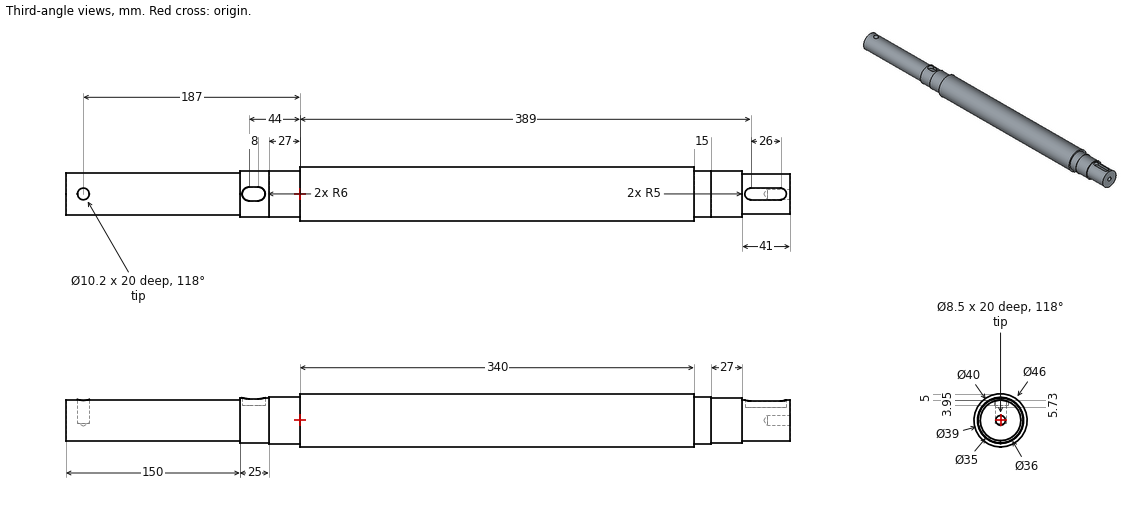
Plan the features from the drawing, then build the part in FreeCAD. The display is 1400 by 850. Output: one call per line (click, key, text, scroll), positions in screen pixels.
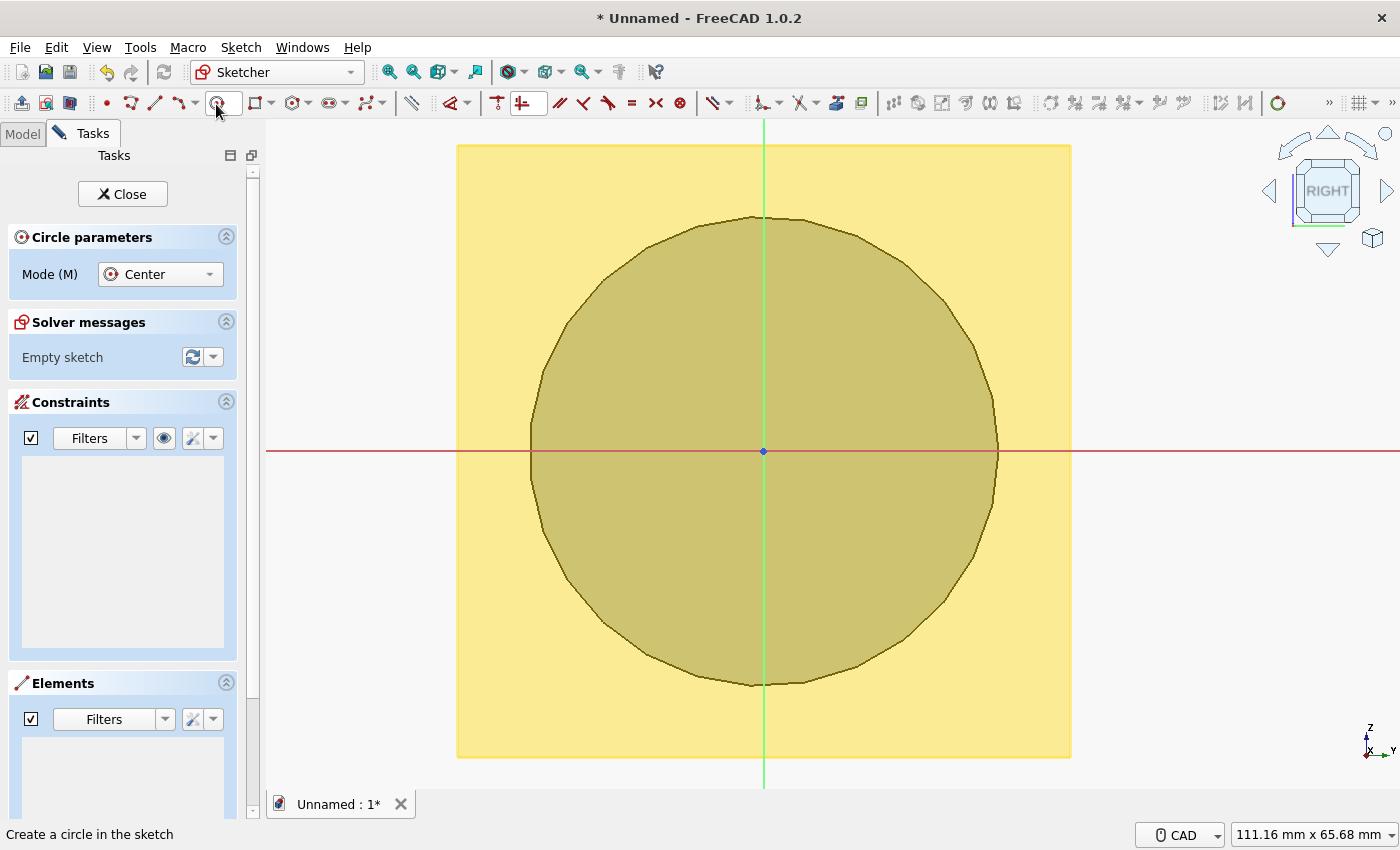
click(764, 451)
click(908, 307)
key(Escape)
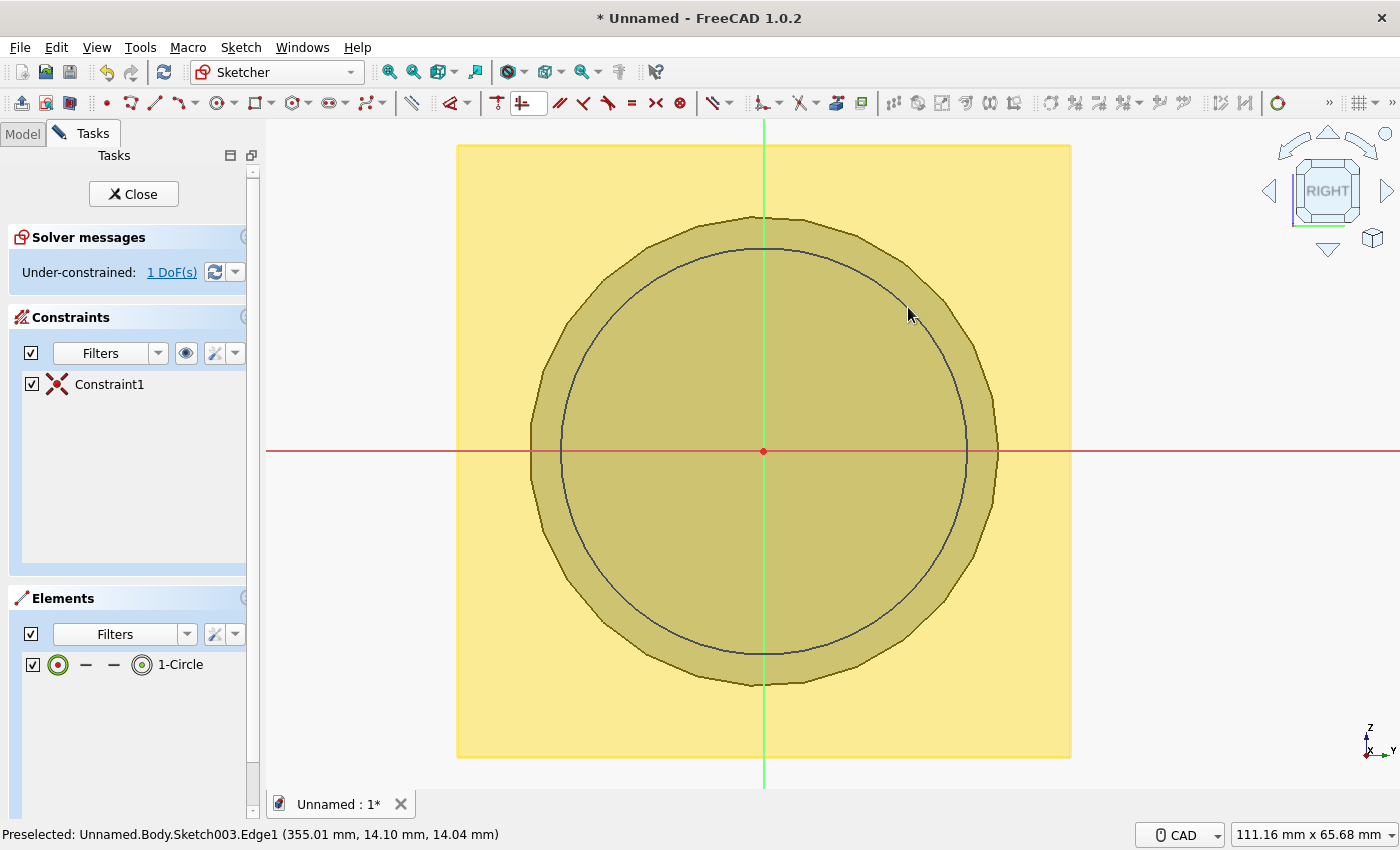
click(450, 104)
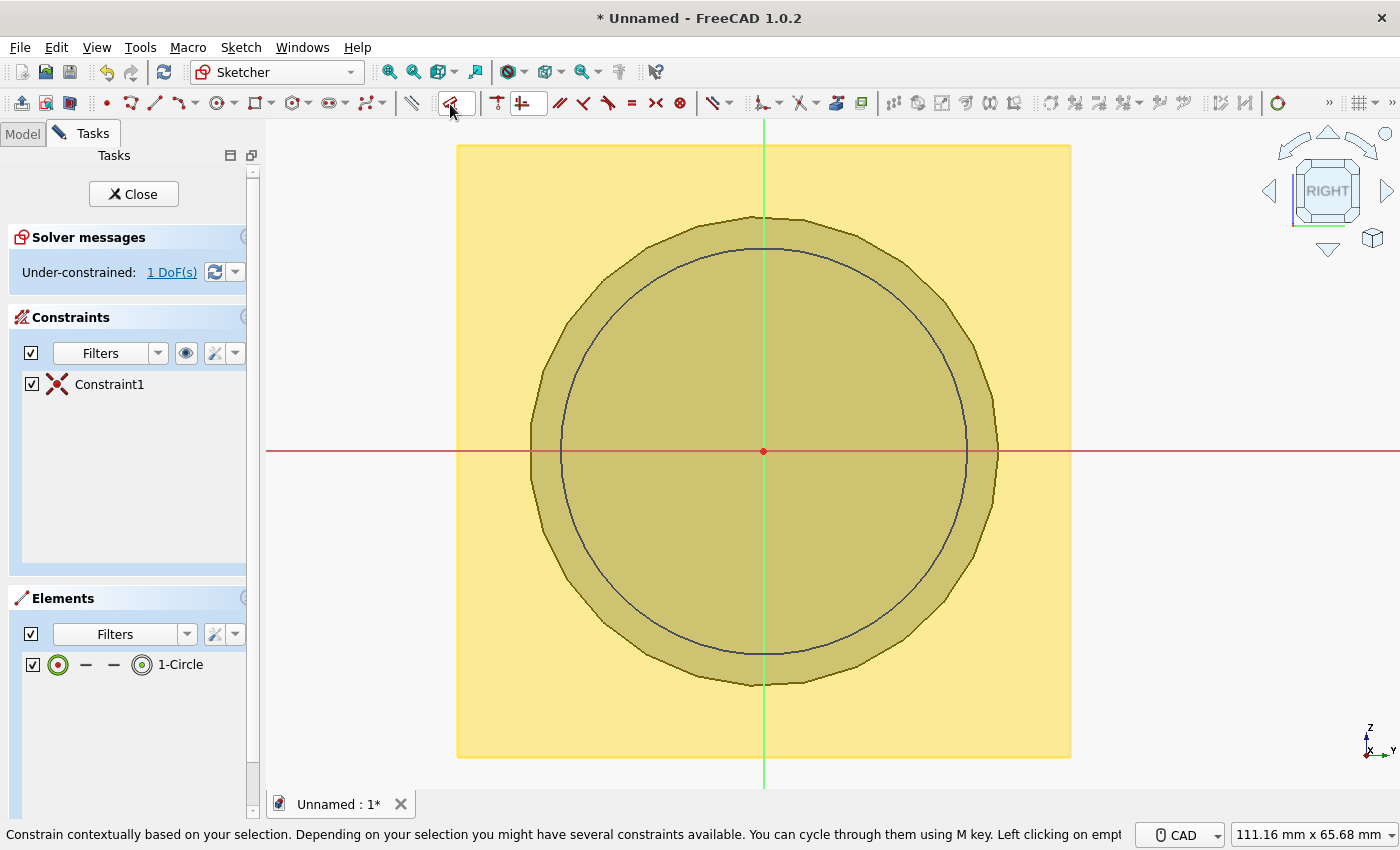
click(907, 307)
click(930, 284)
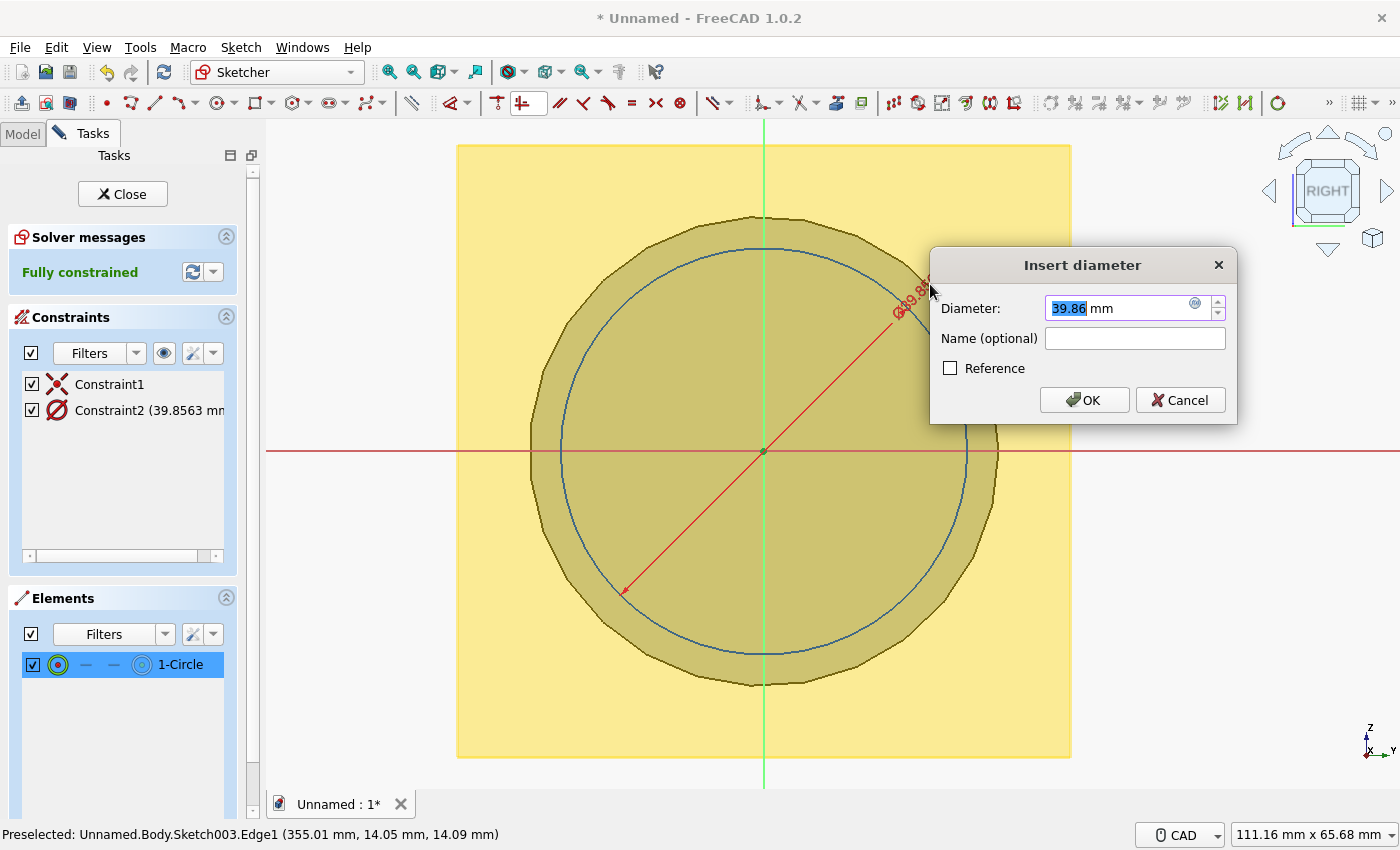
text(40)
key(Return)
key(Escape)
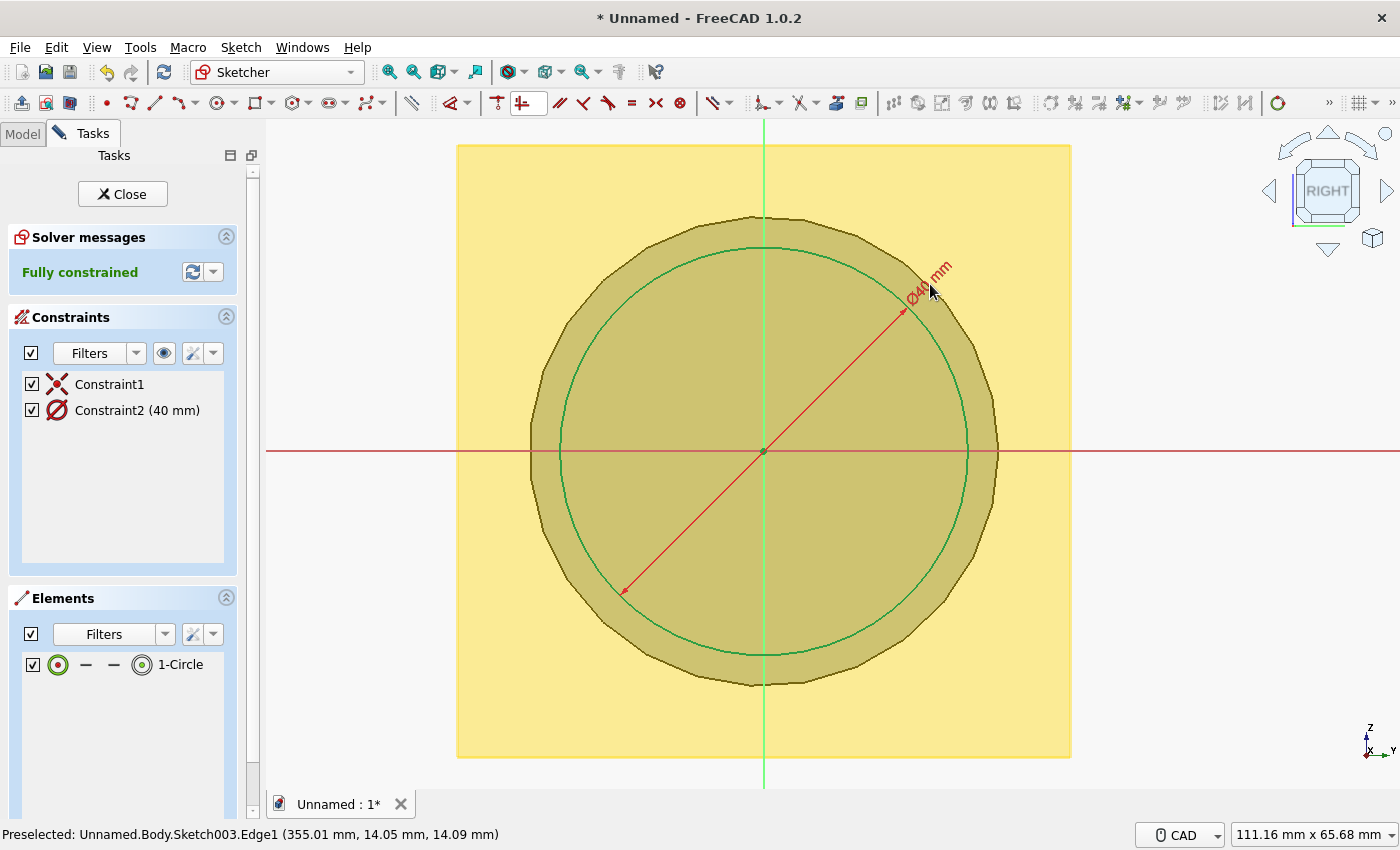
click(123, 194)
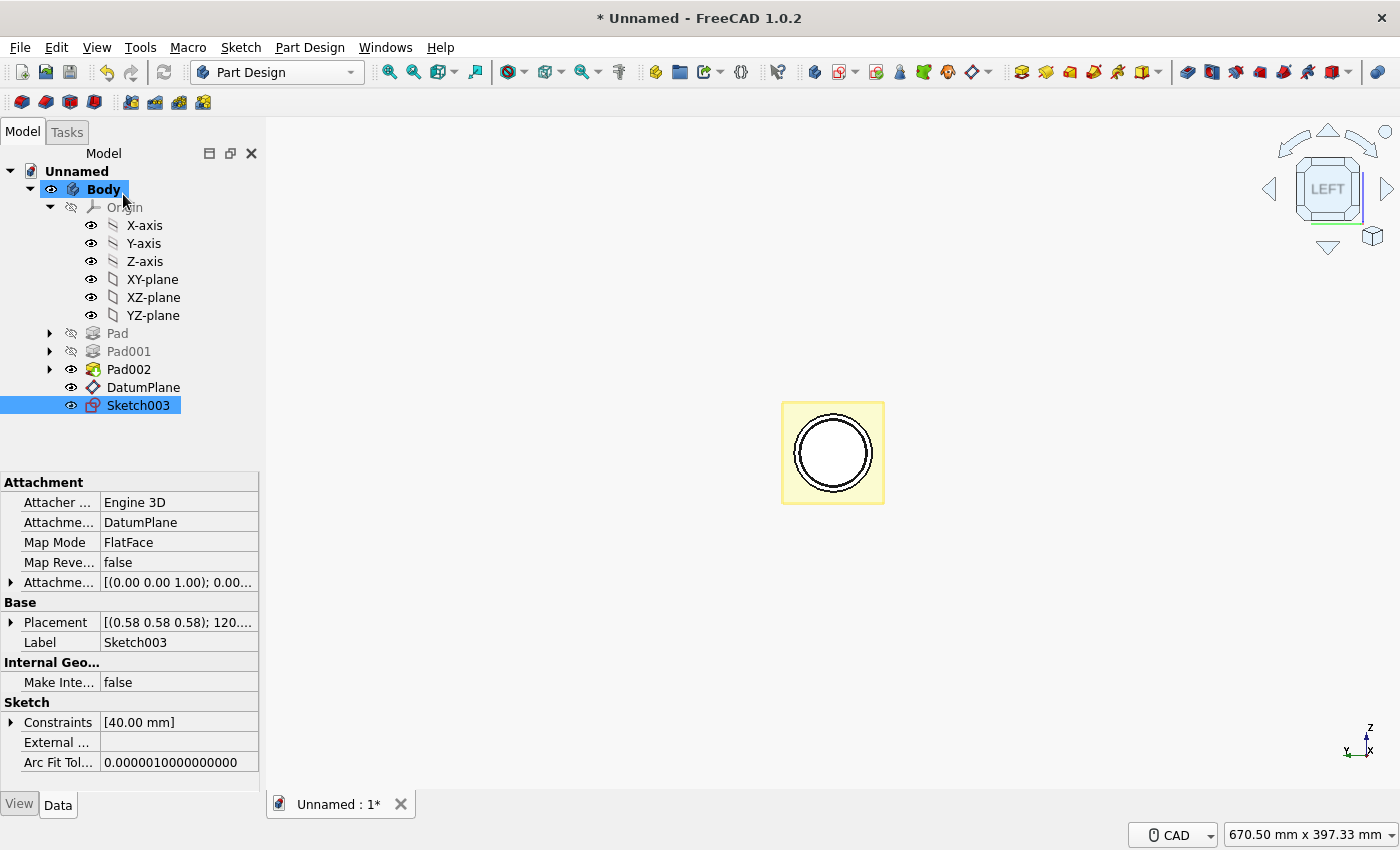
click(1022, 72)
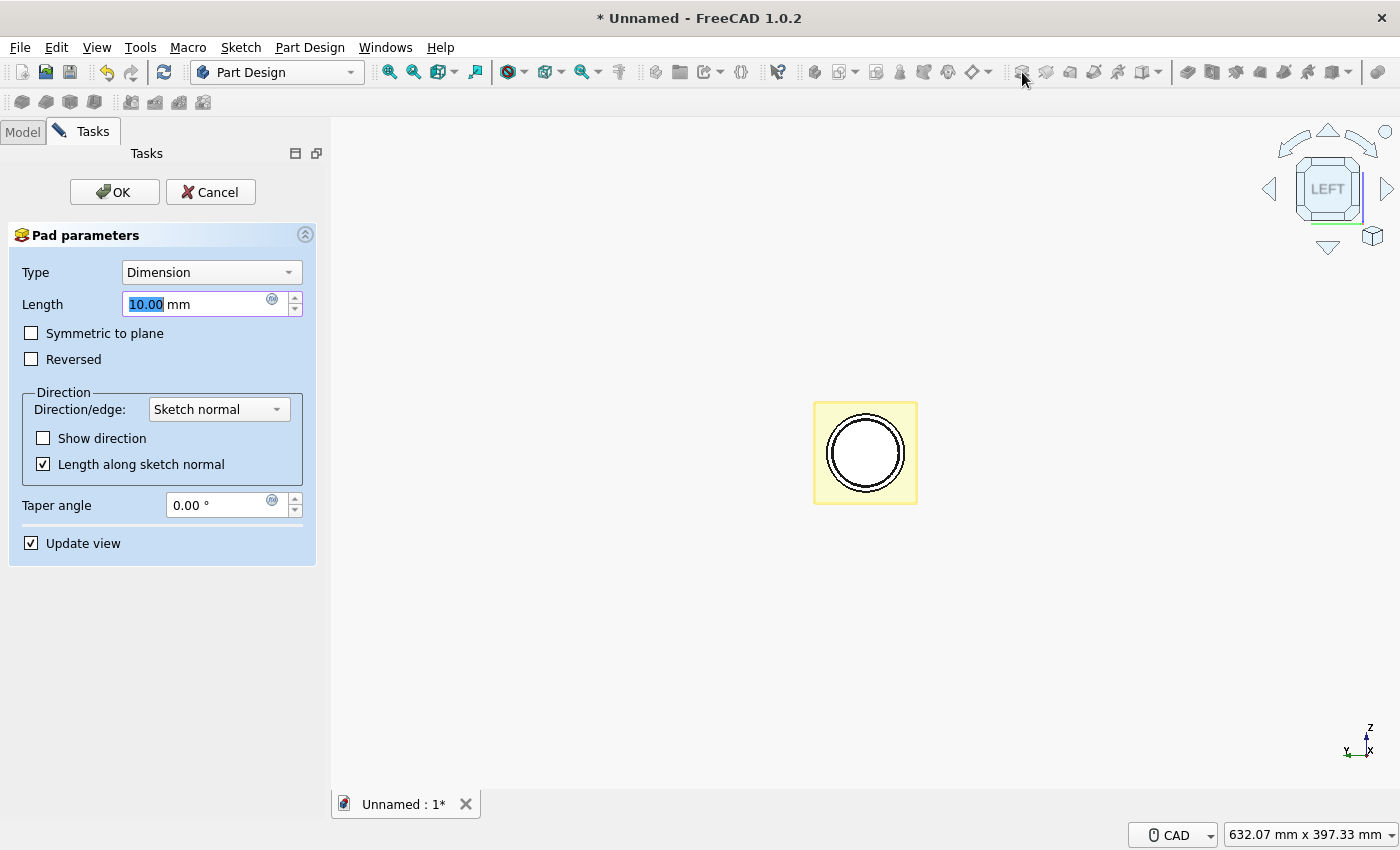
text(15)
key(Tab)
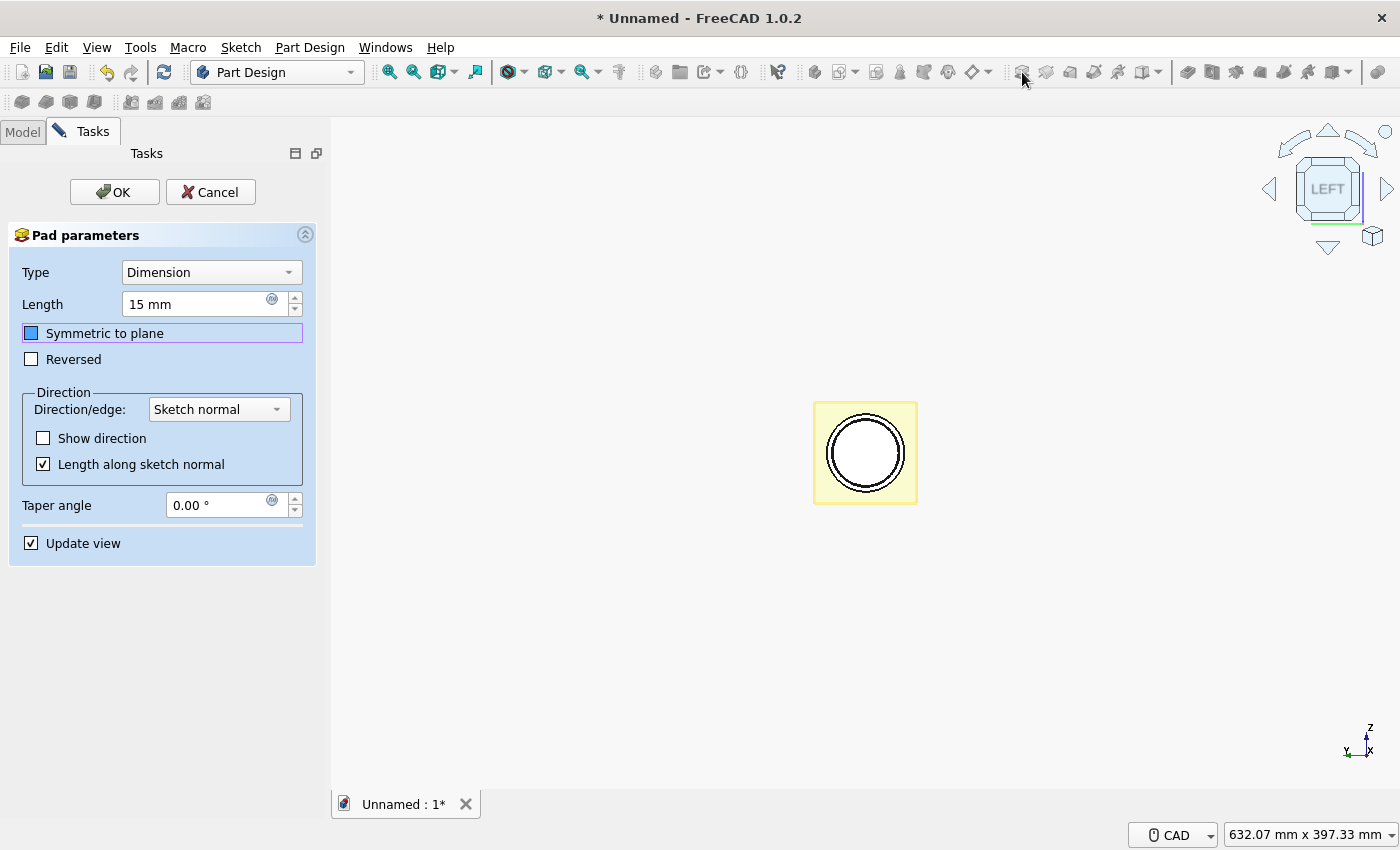
click(30, 359)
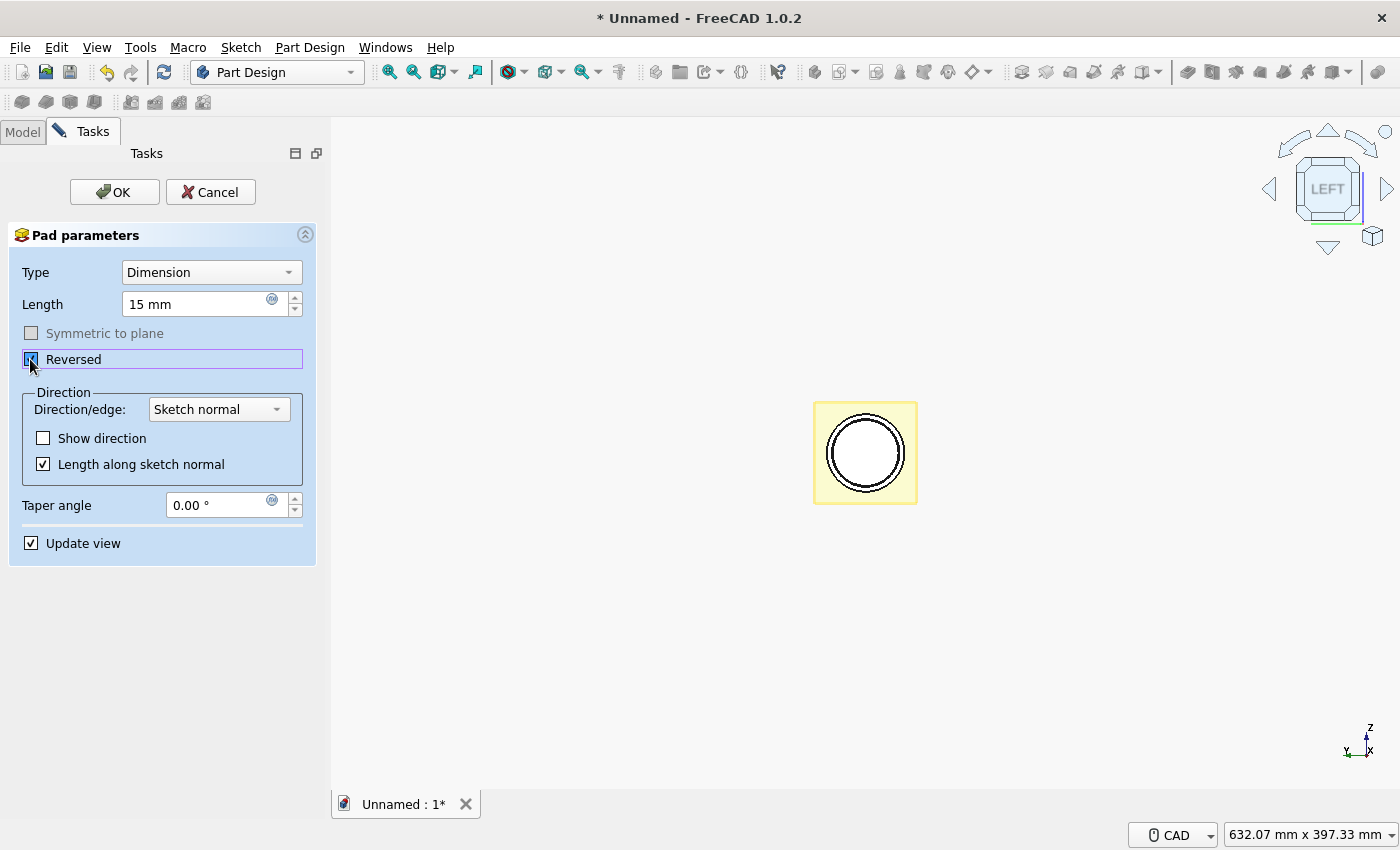
click(115, 192)